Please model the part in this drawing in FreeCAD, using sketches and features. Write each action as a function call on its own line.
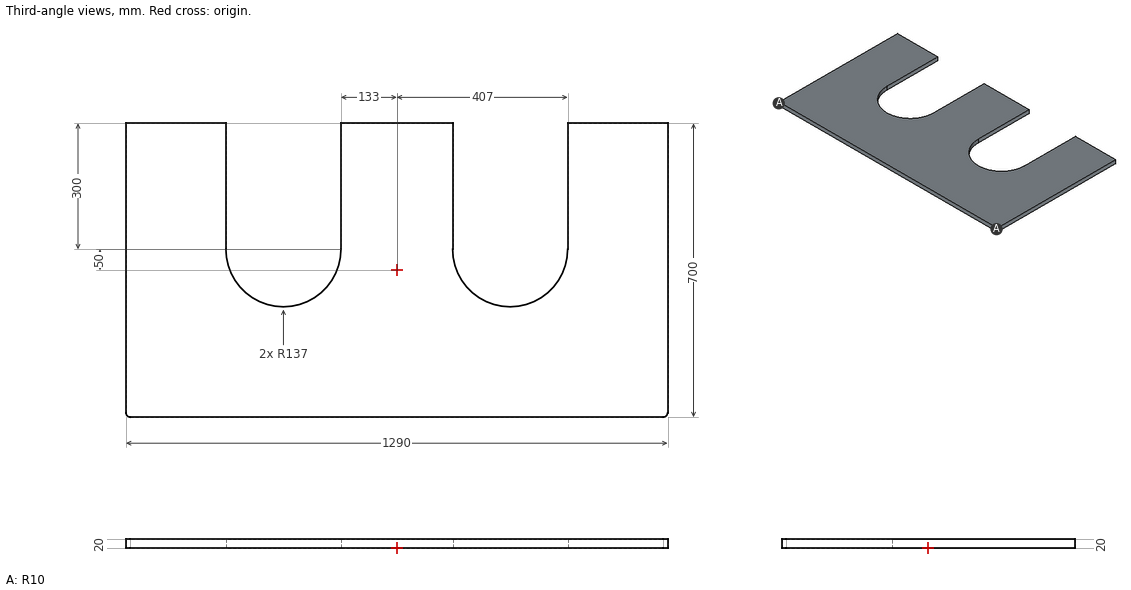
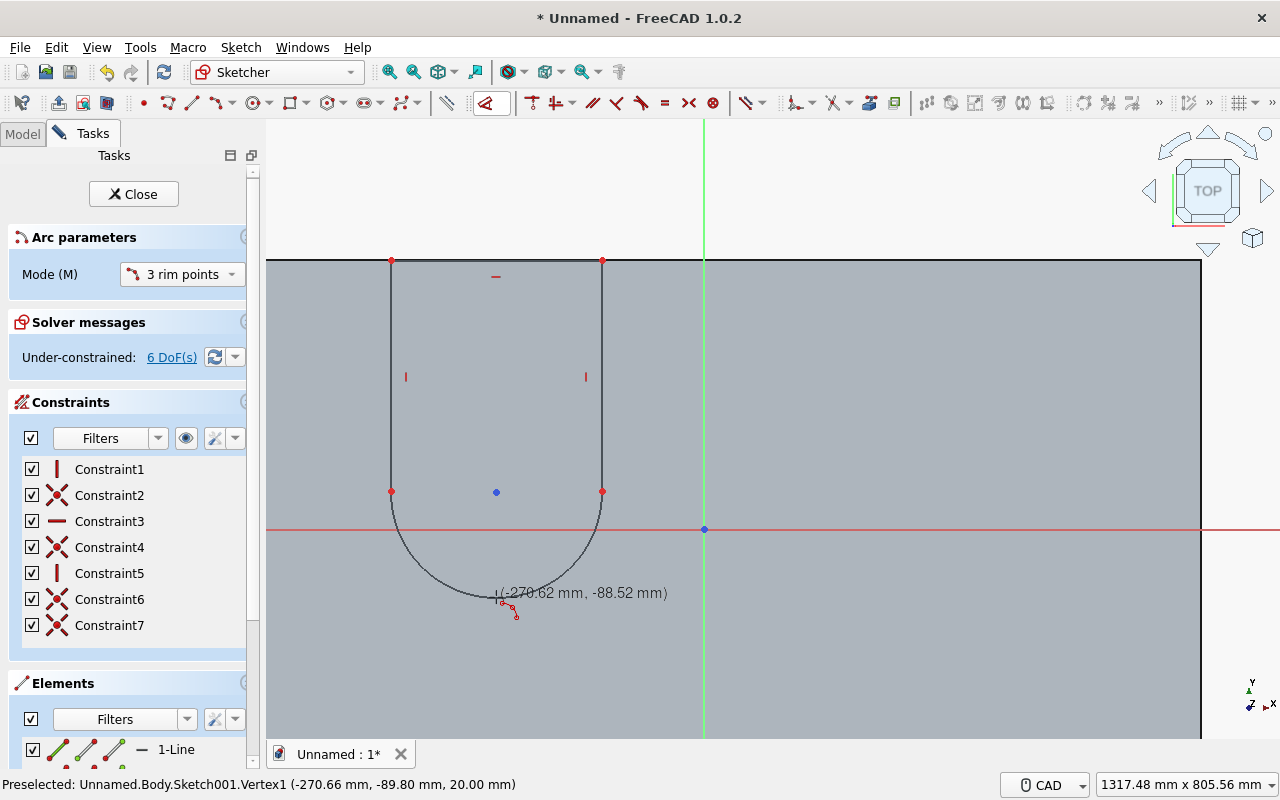
click(168, 104)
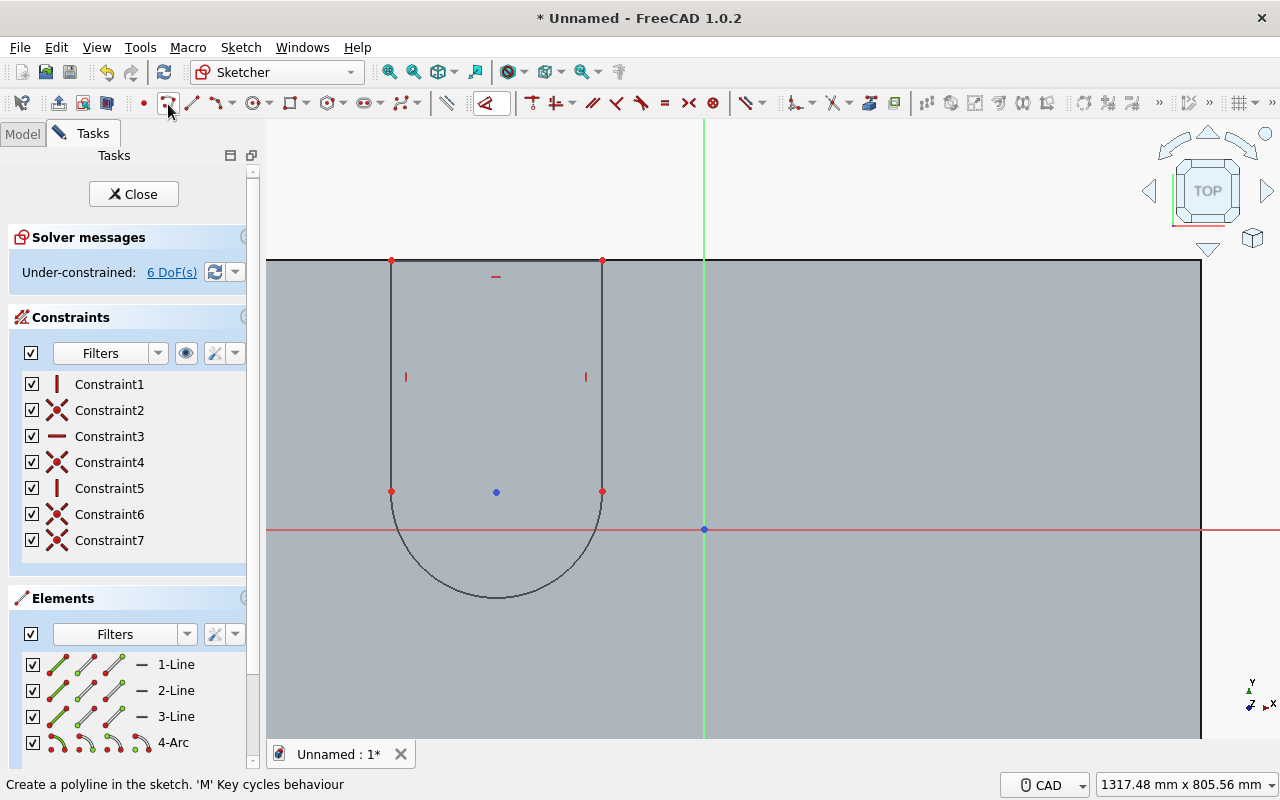
click(1018, 491)
click(1018, 260)
click(807, 260)
click(807, 491)
right_click(807, 491)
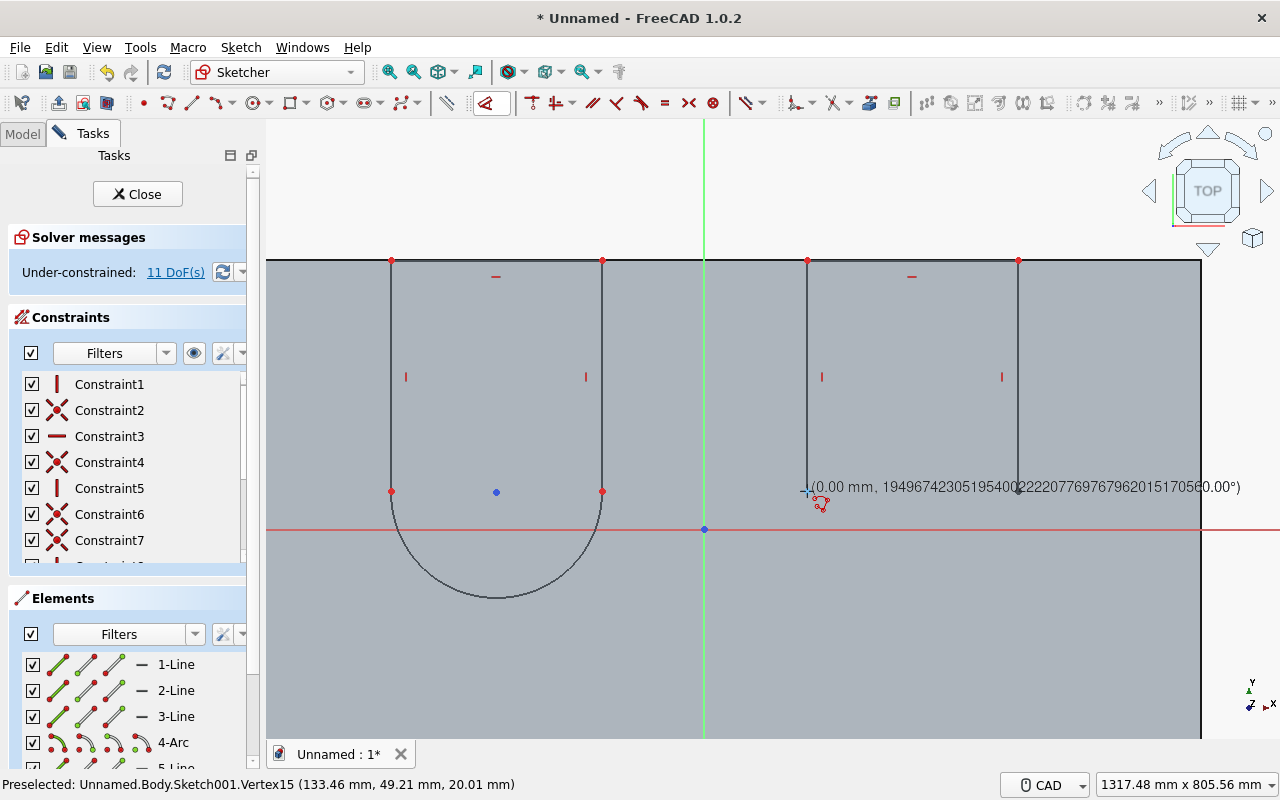
key(g)
key(3)
key(a)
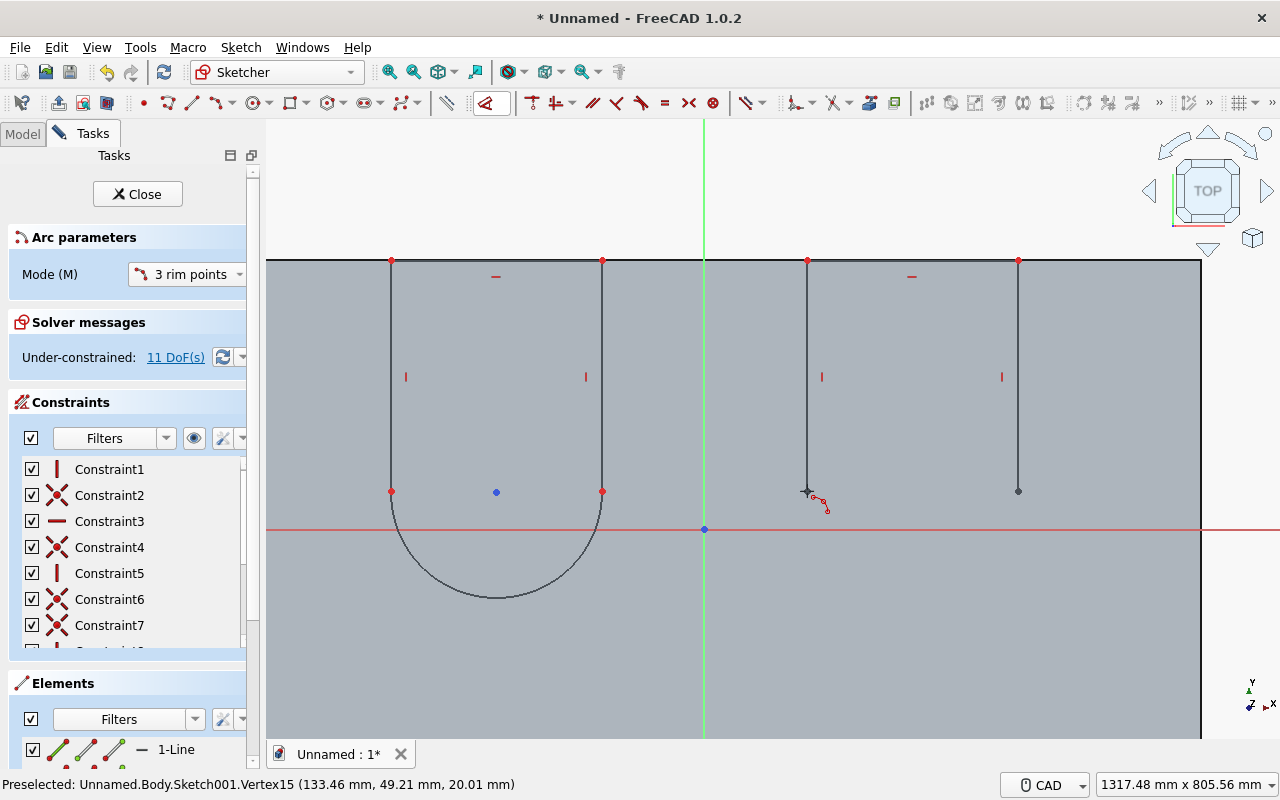
click(807, 492)
click(1018, 492)
click(912, 597)
key(Escape)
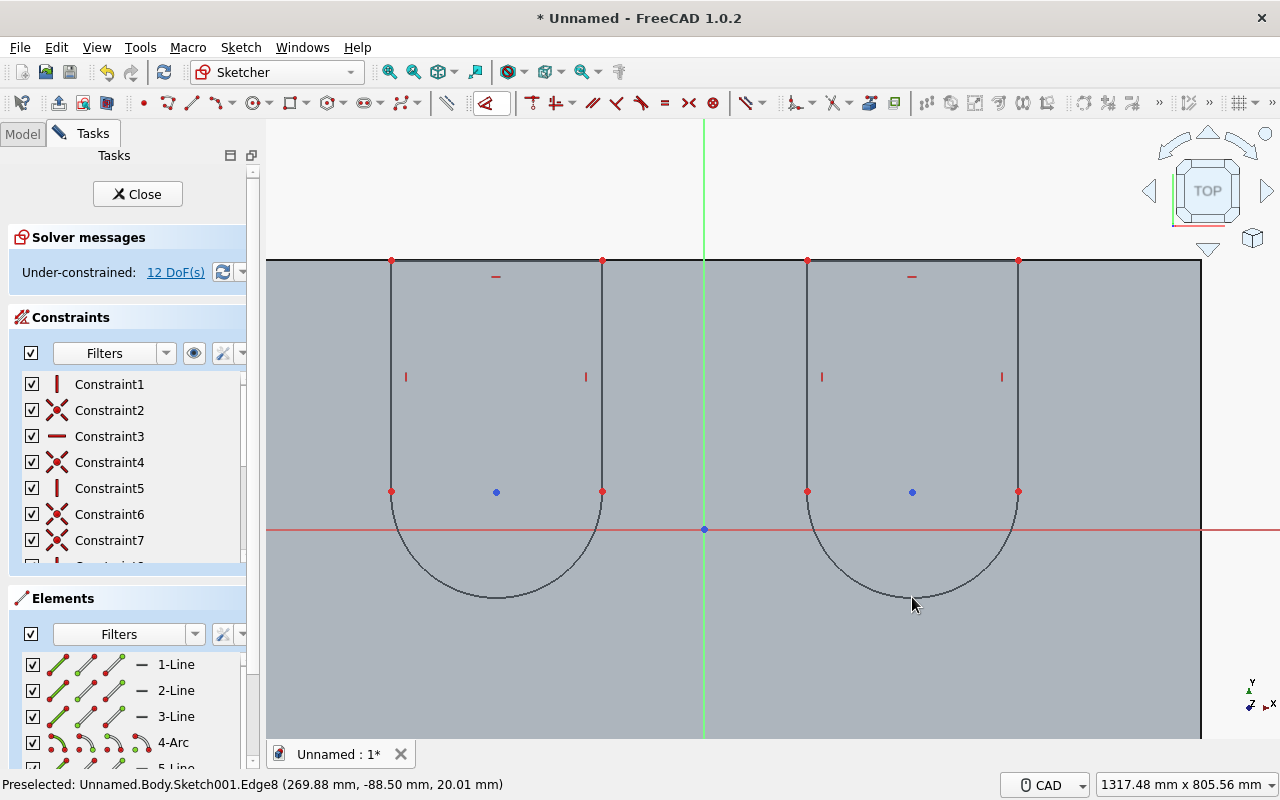
click(434, 578)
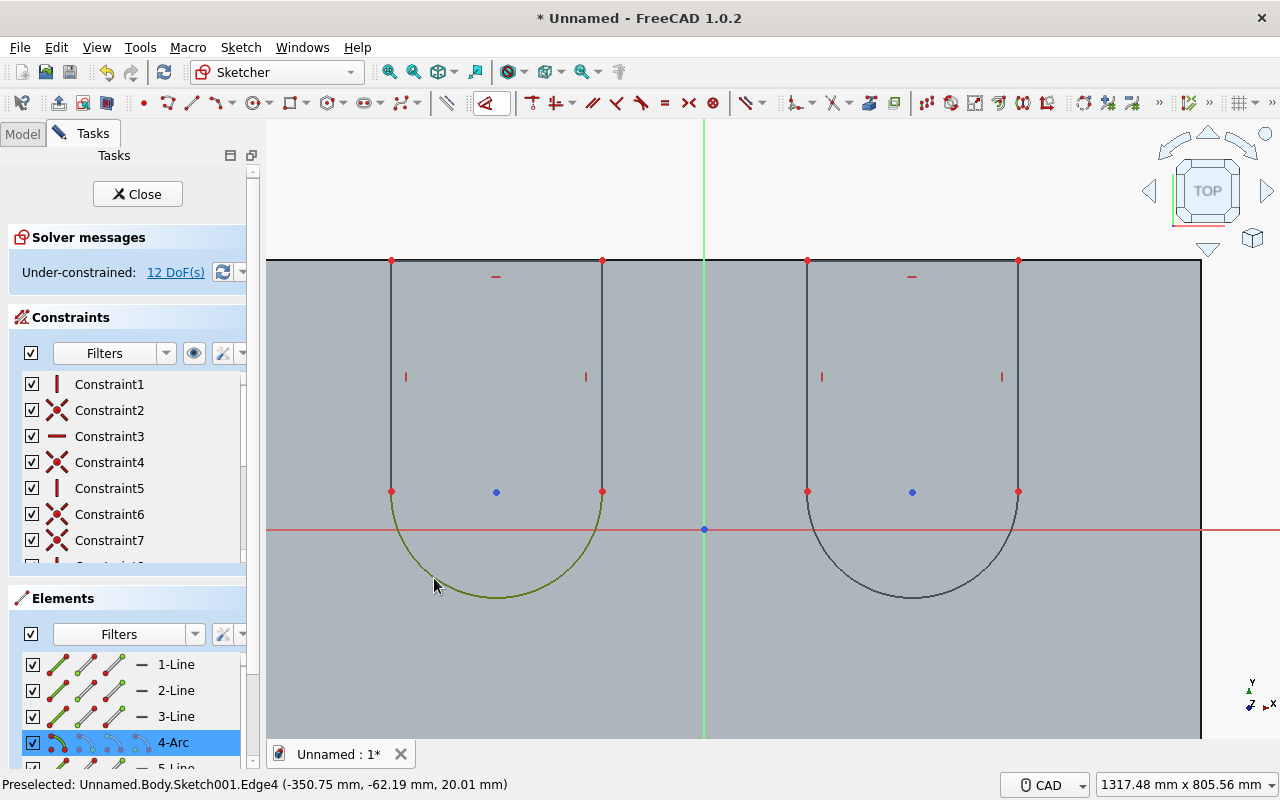
click(850, 578)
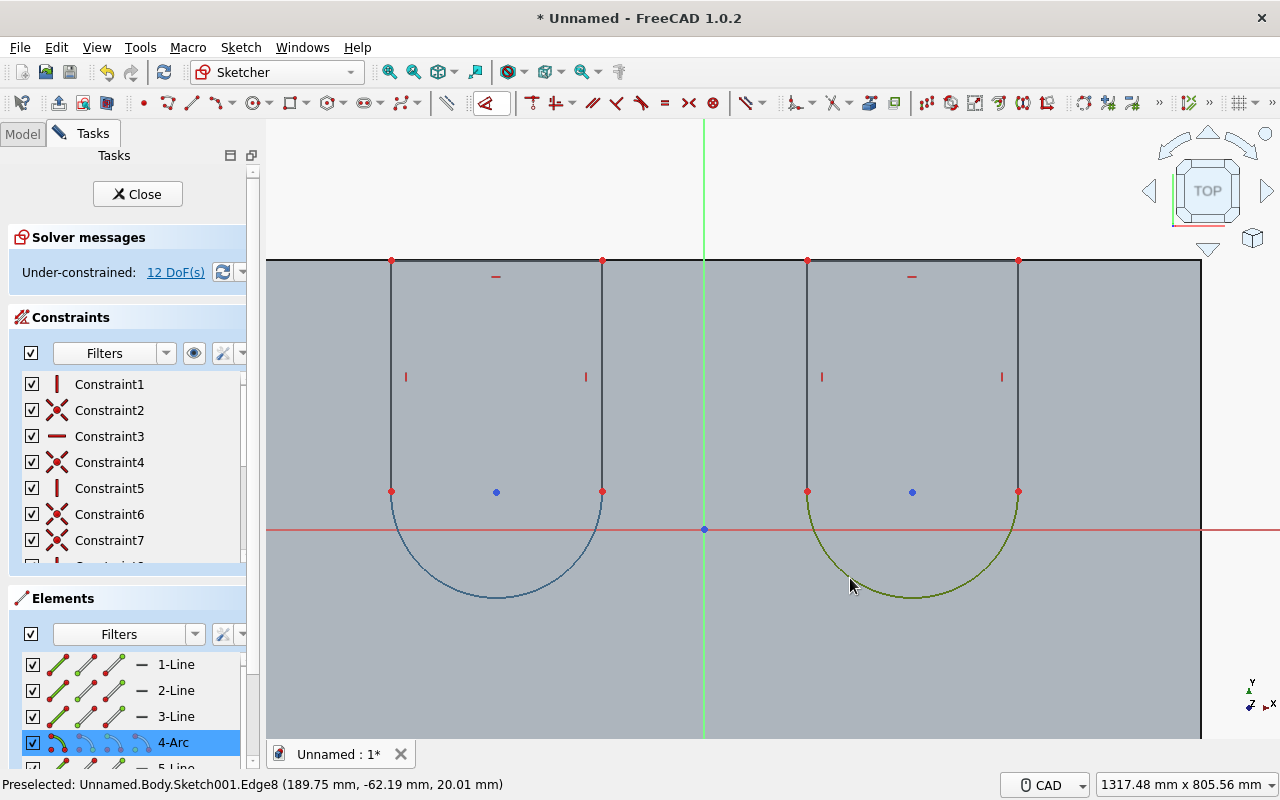
key(e)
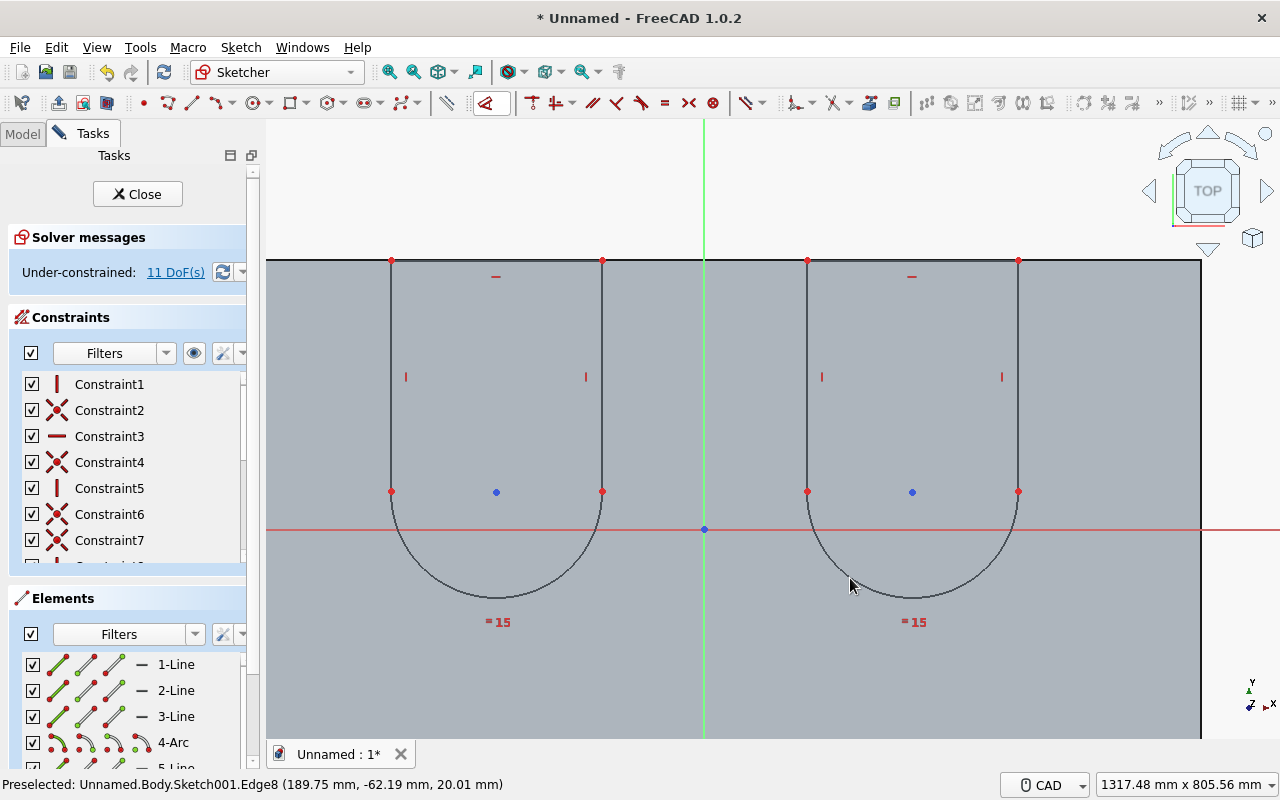
click(486, 104)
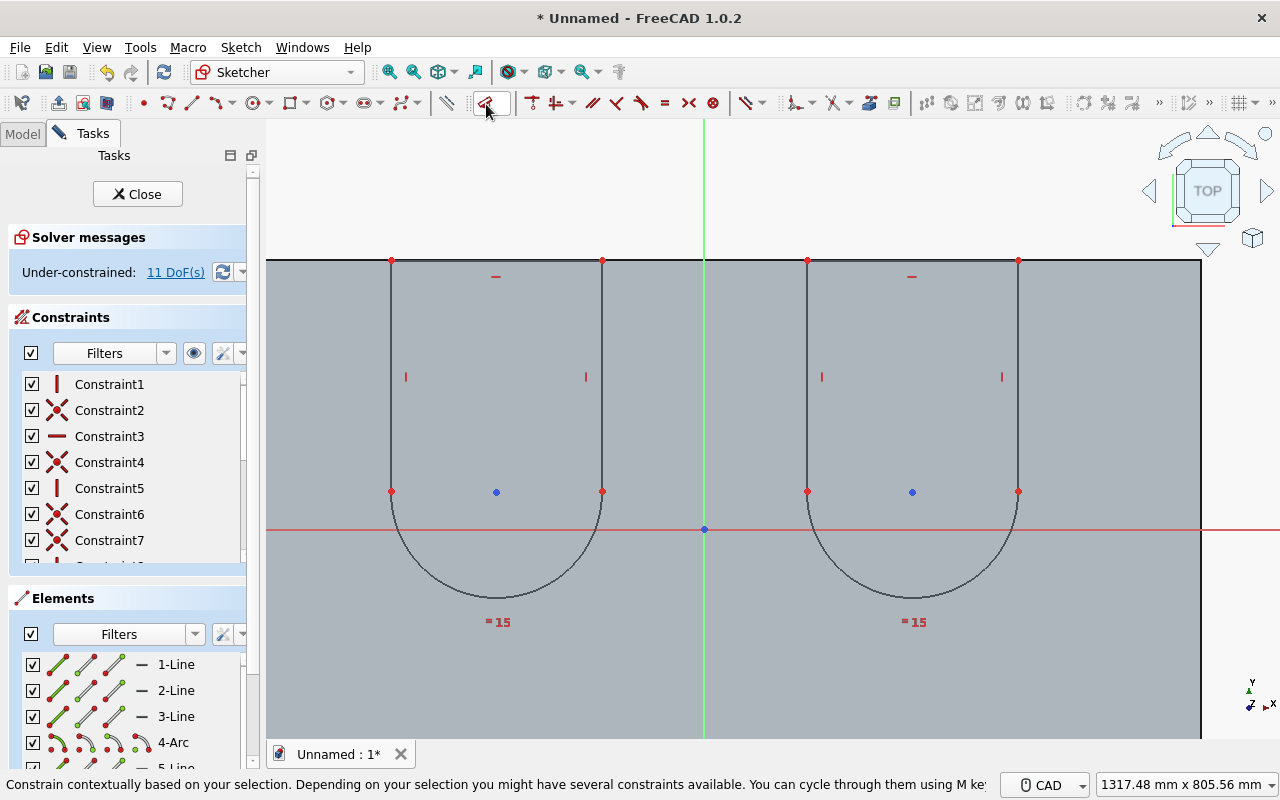
click(434, 578)
click(415, 604)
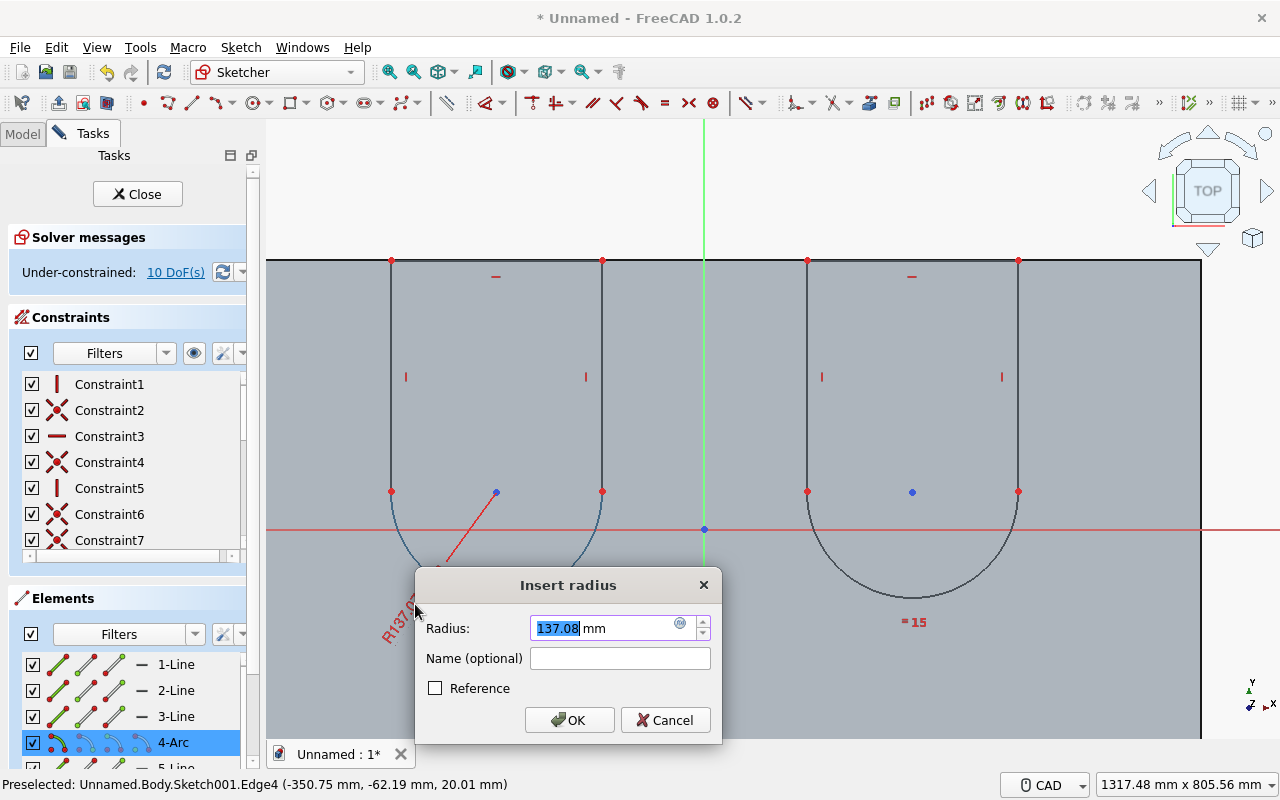
text(137)
key(Return)